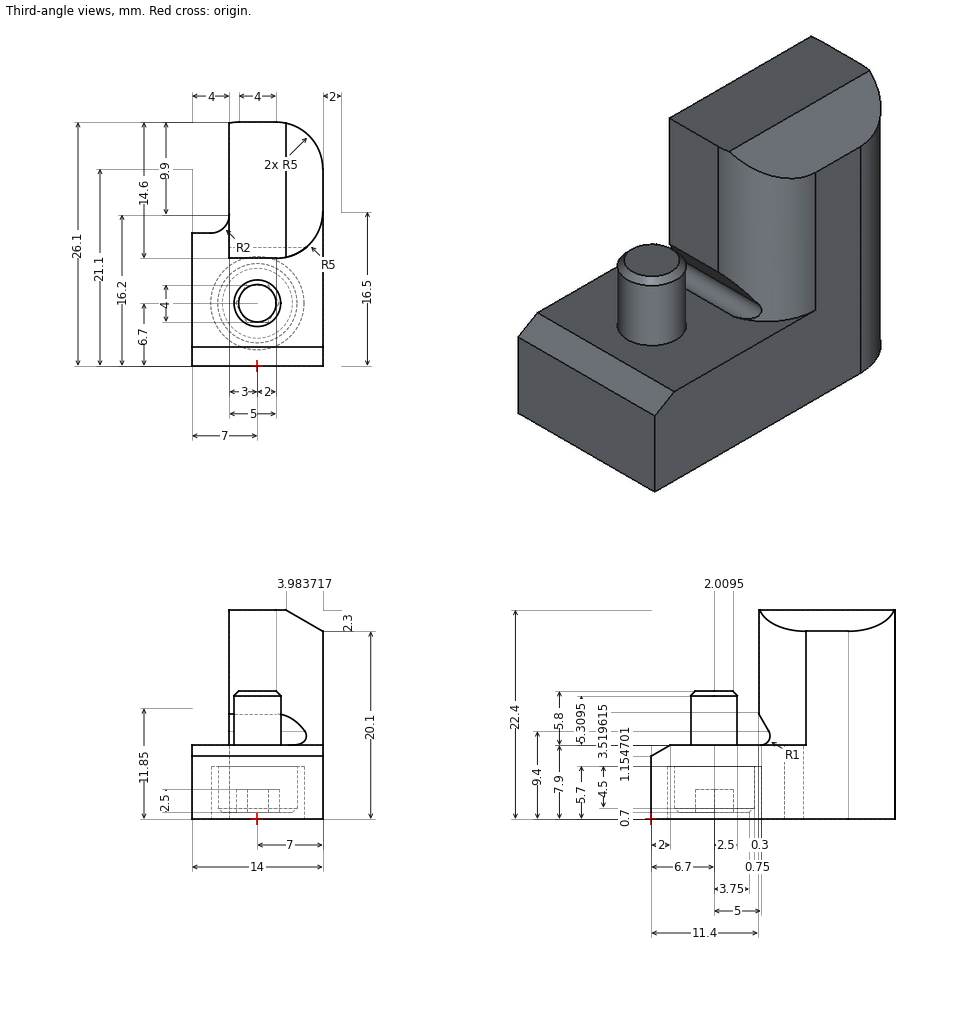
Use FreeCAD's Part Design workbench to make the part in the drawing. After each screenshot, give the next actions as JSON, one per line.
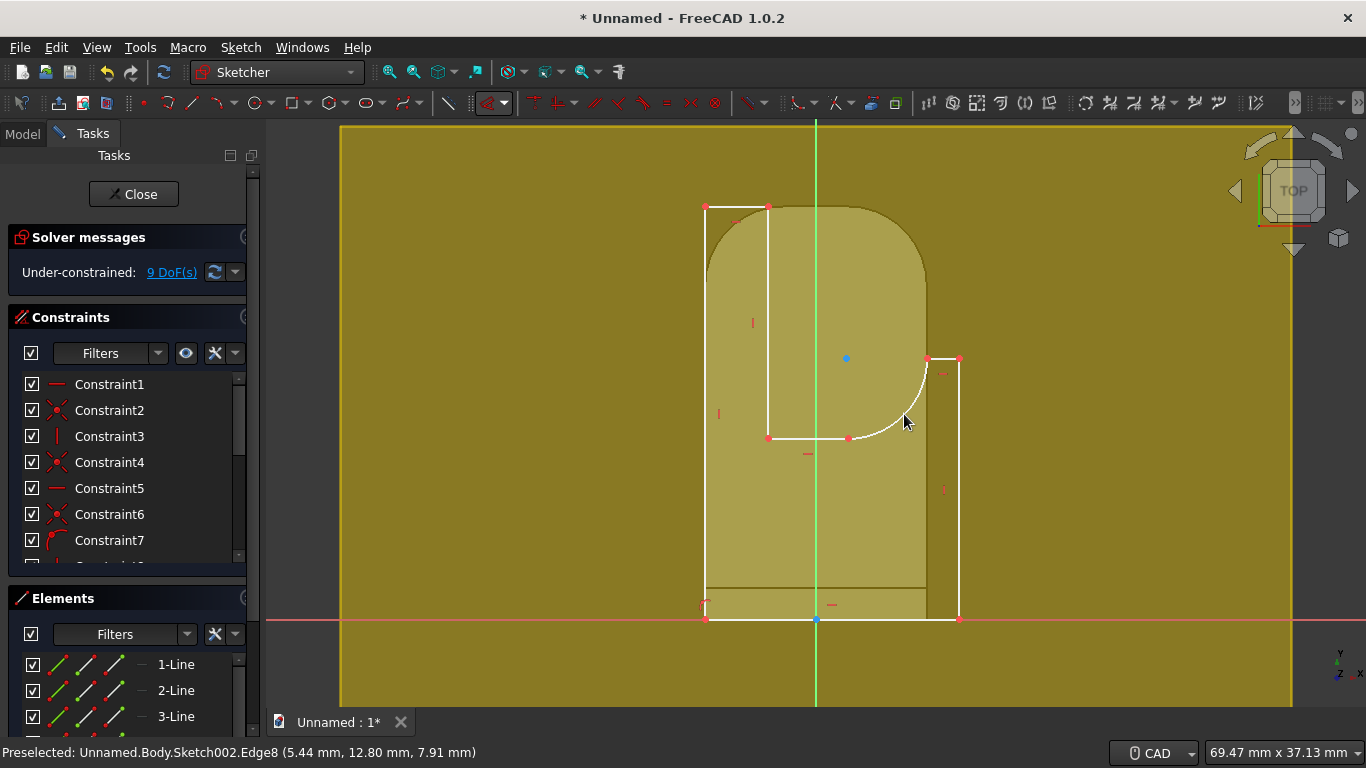
{"action": "left_click", "coordinate": [792, 439]}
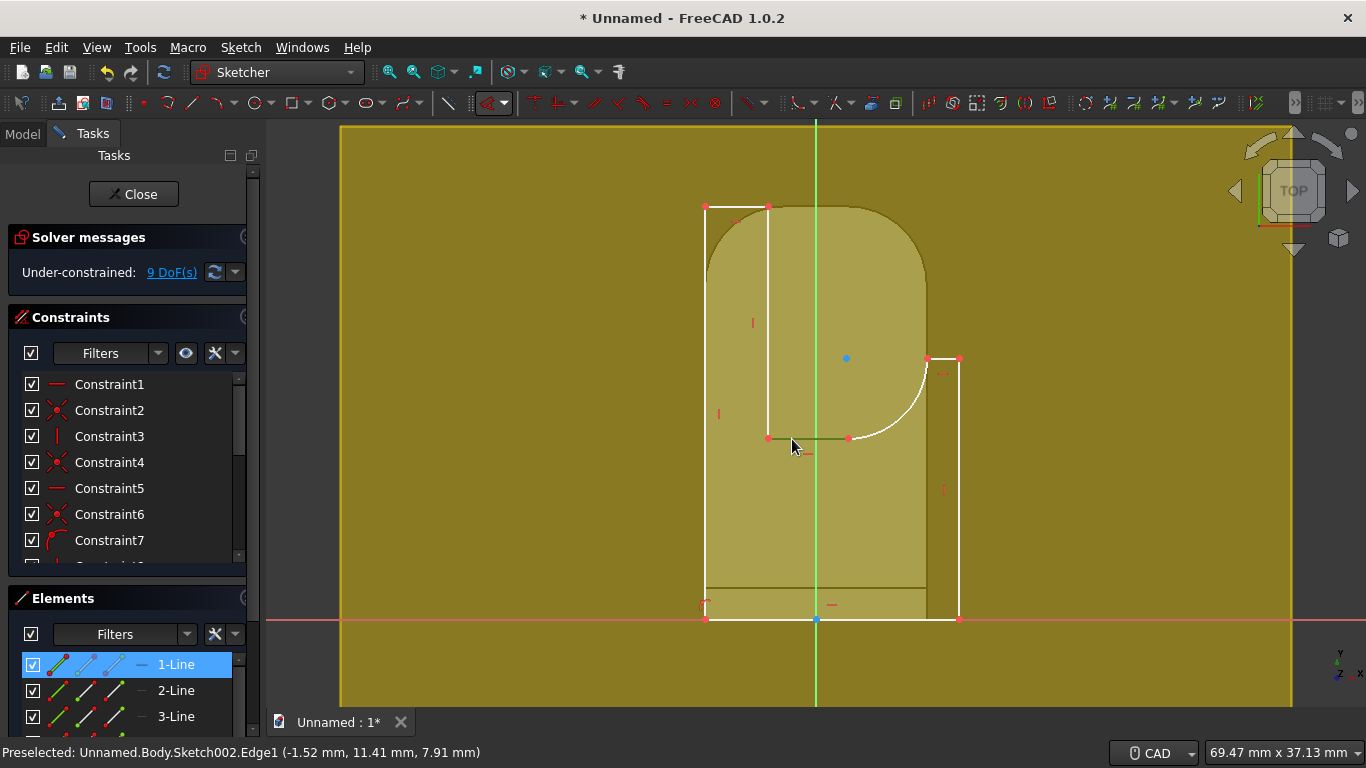
{"action": "left_click", "coordinate": [884, 430]}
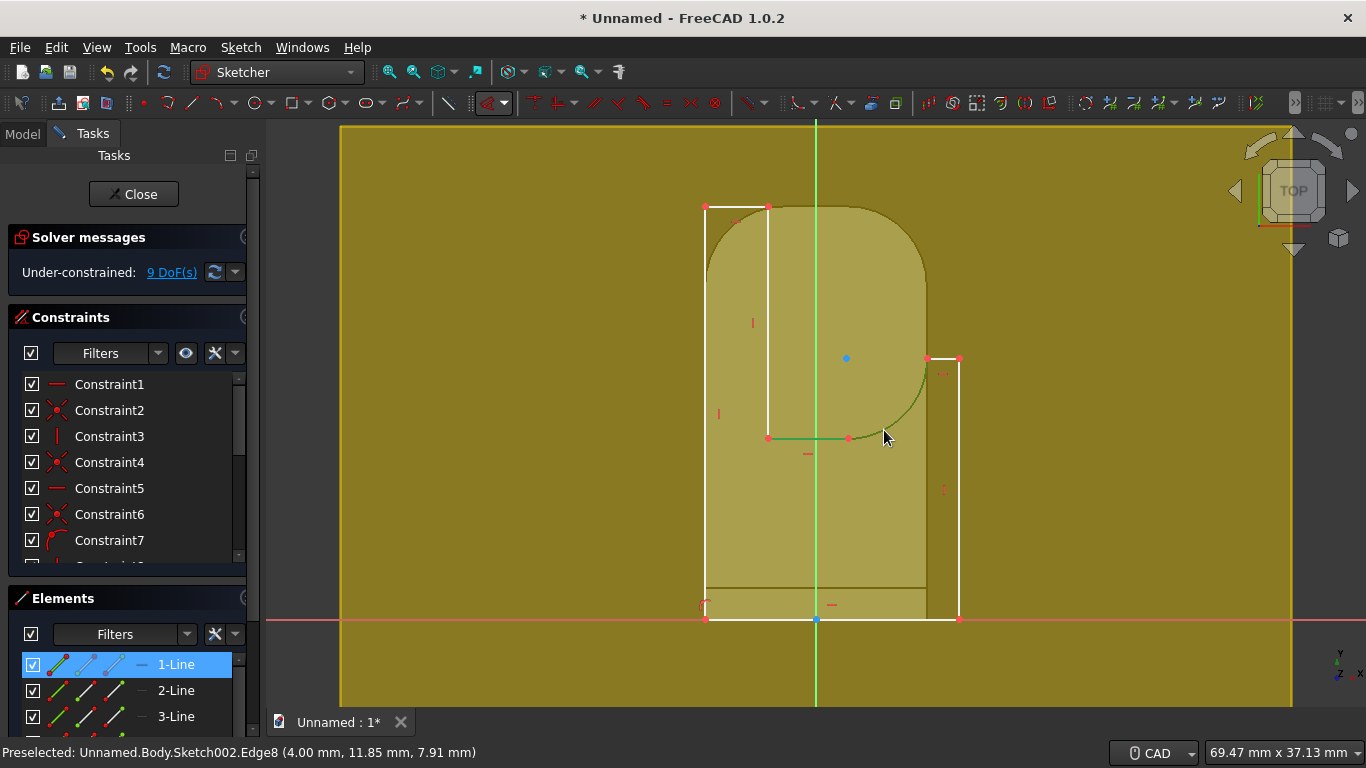
{"action": "left_click", "coordinate": [644, 104]}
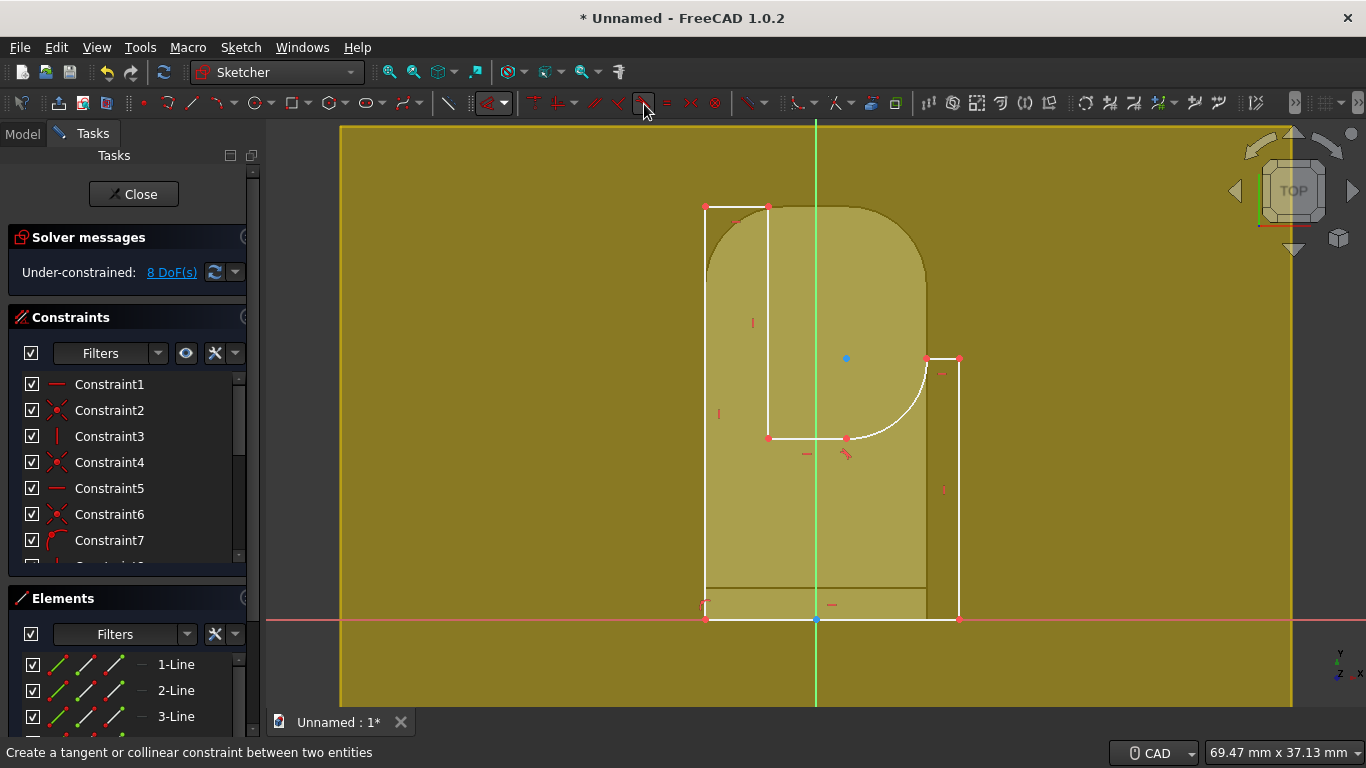
{"action": "left_click", "coordinate": [883, 430]}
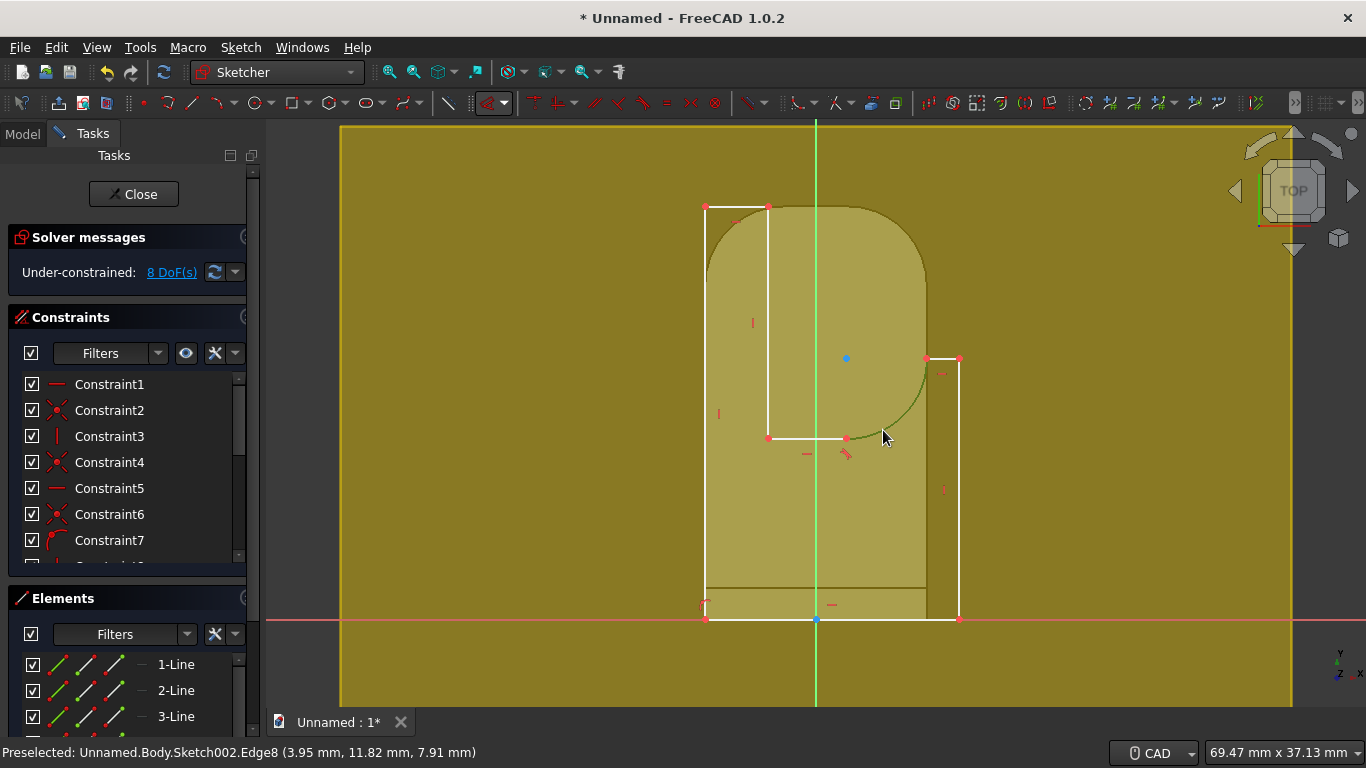
{"action": "left_click", "coordinate": [506, 104]}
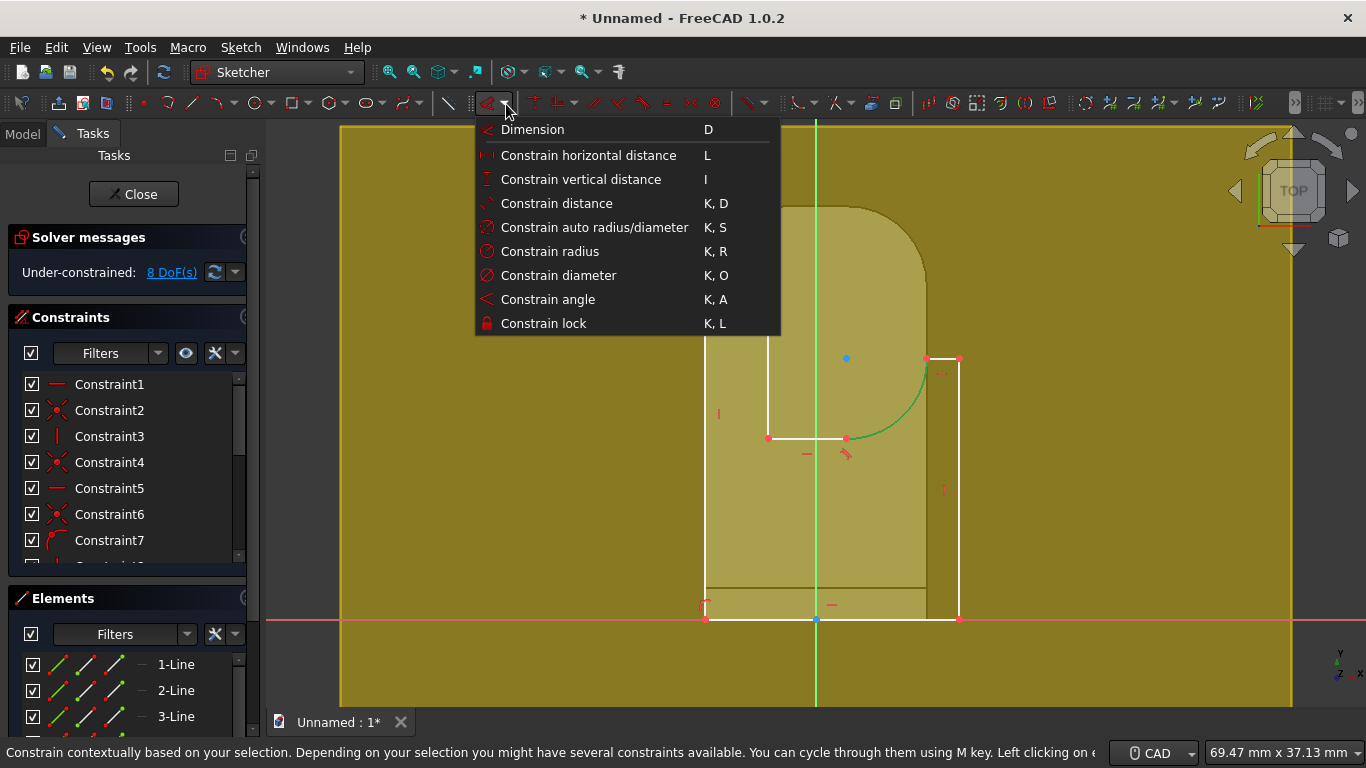
{"action": "left_click", "coordinate": [628, 251]}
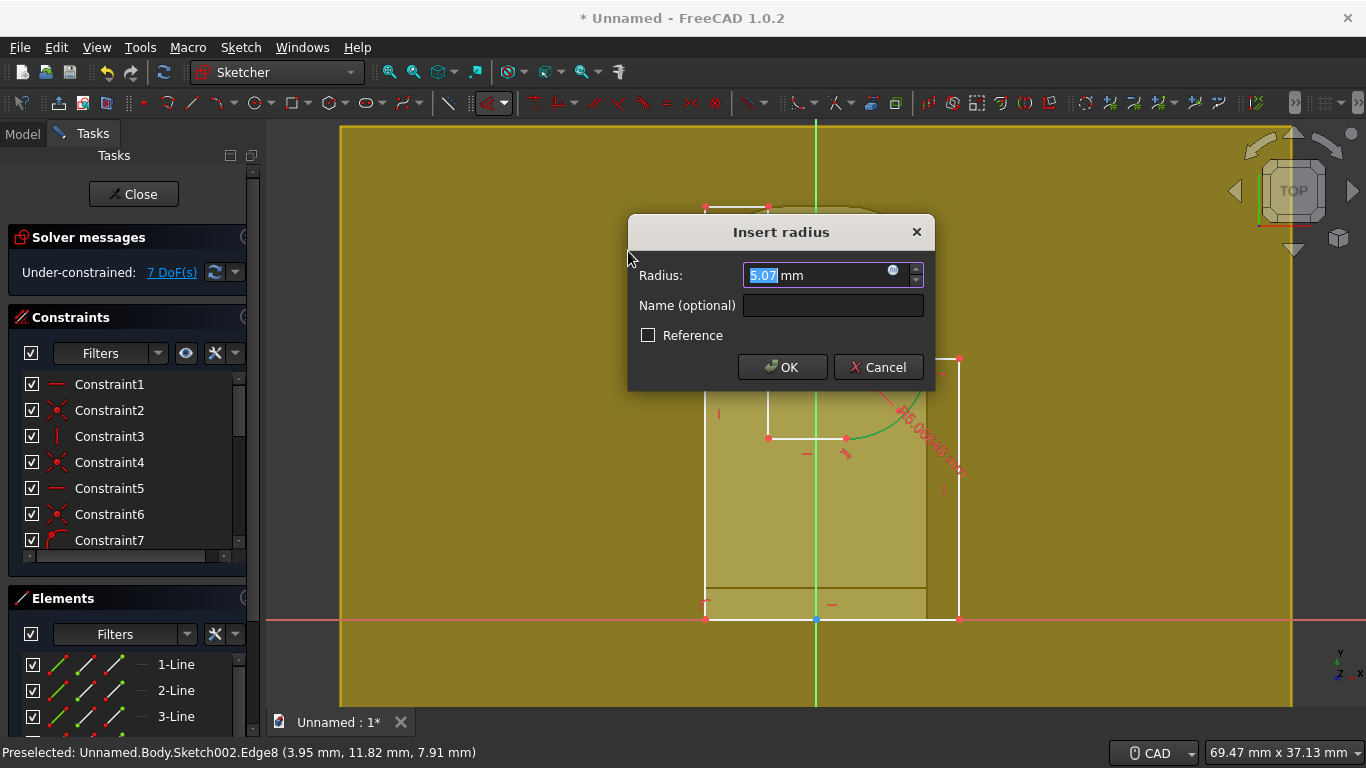
{"action": "type", "text": "5"}
{"action": "key", "text": "Return"}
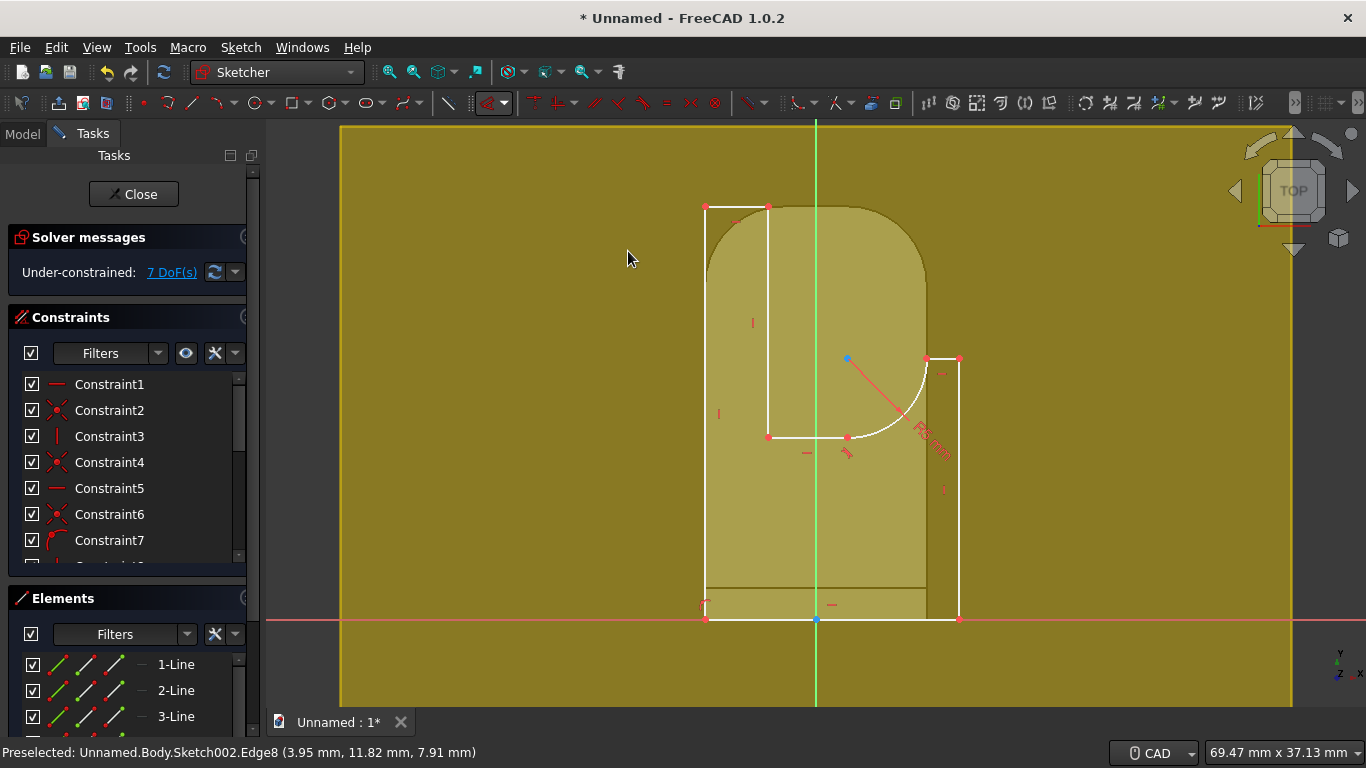
{"action": "left_click", "coordinate": [792, 438]}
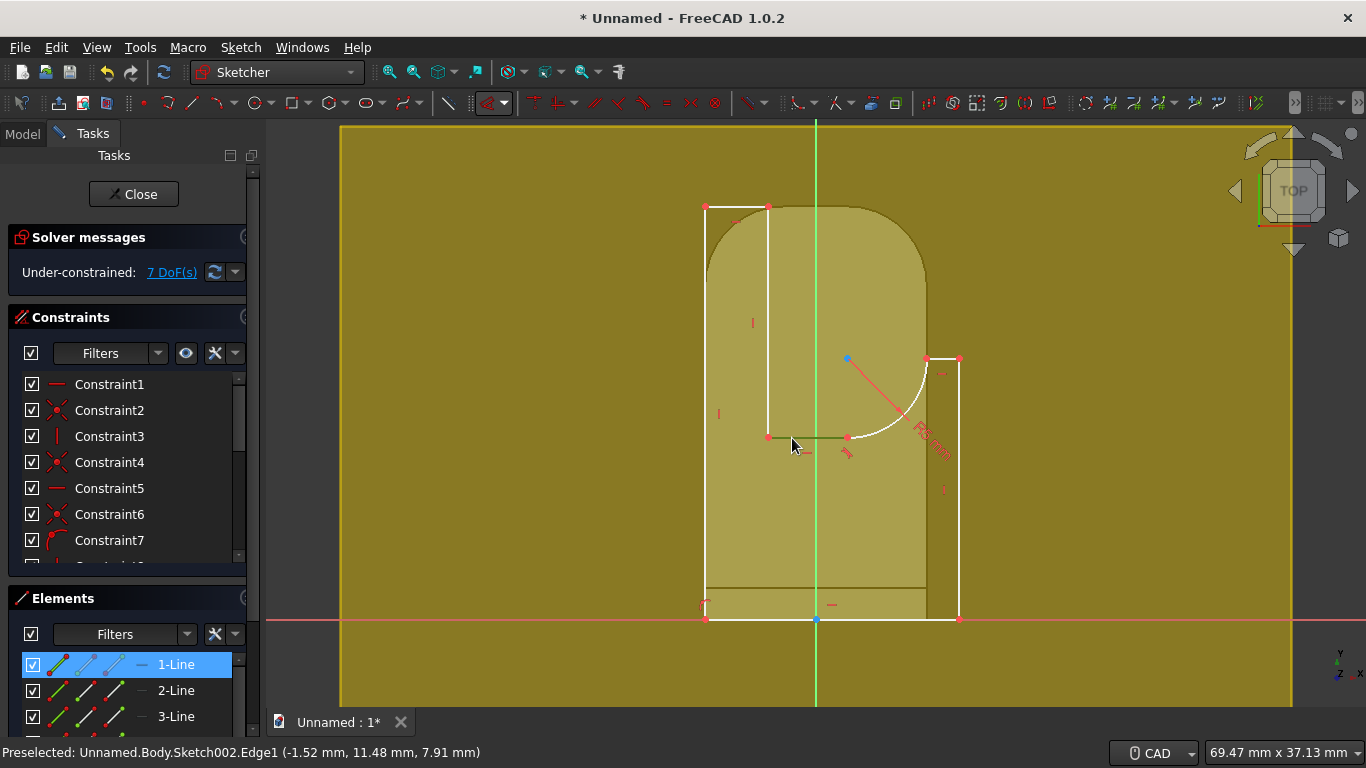
{"action": "left_click", "coordinate": [506, 104]}